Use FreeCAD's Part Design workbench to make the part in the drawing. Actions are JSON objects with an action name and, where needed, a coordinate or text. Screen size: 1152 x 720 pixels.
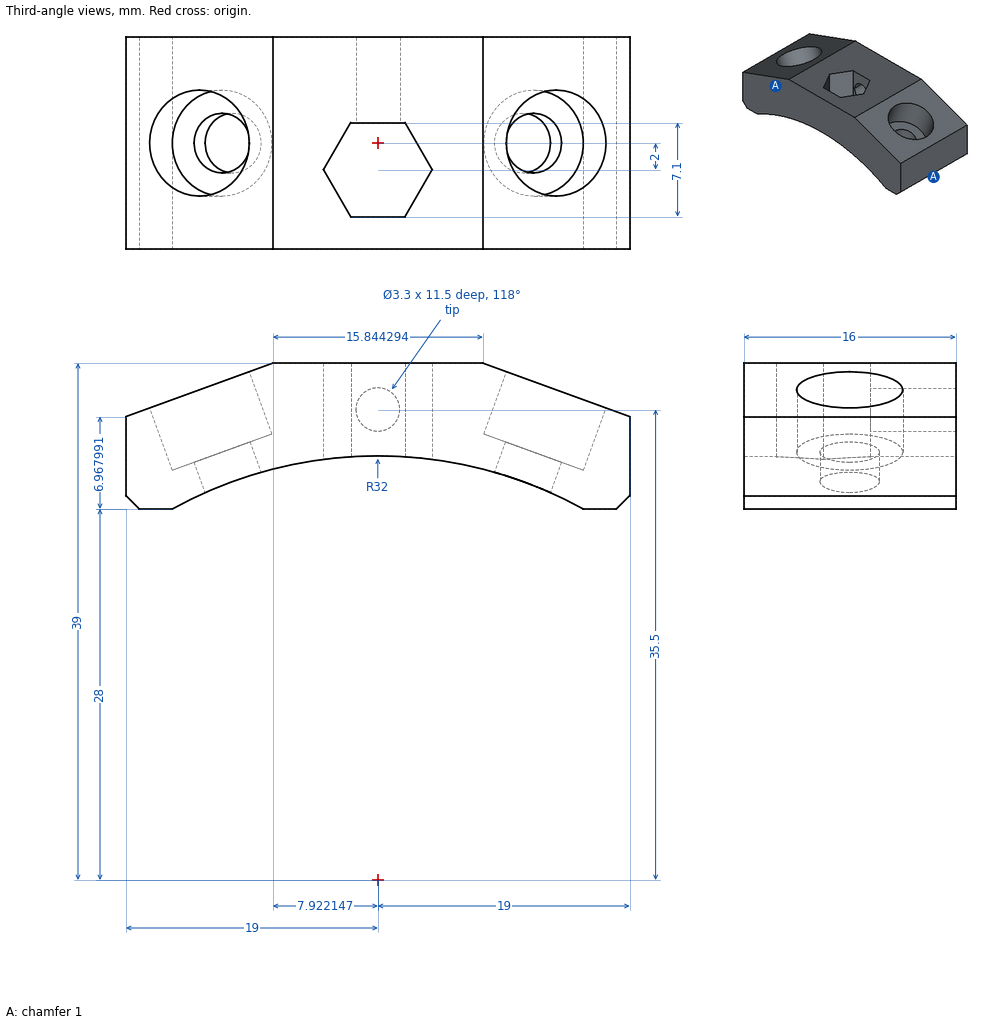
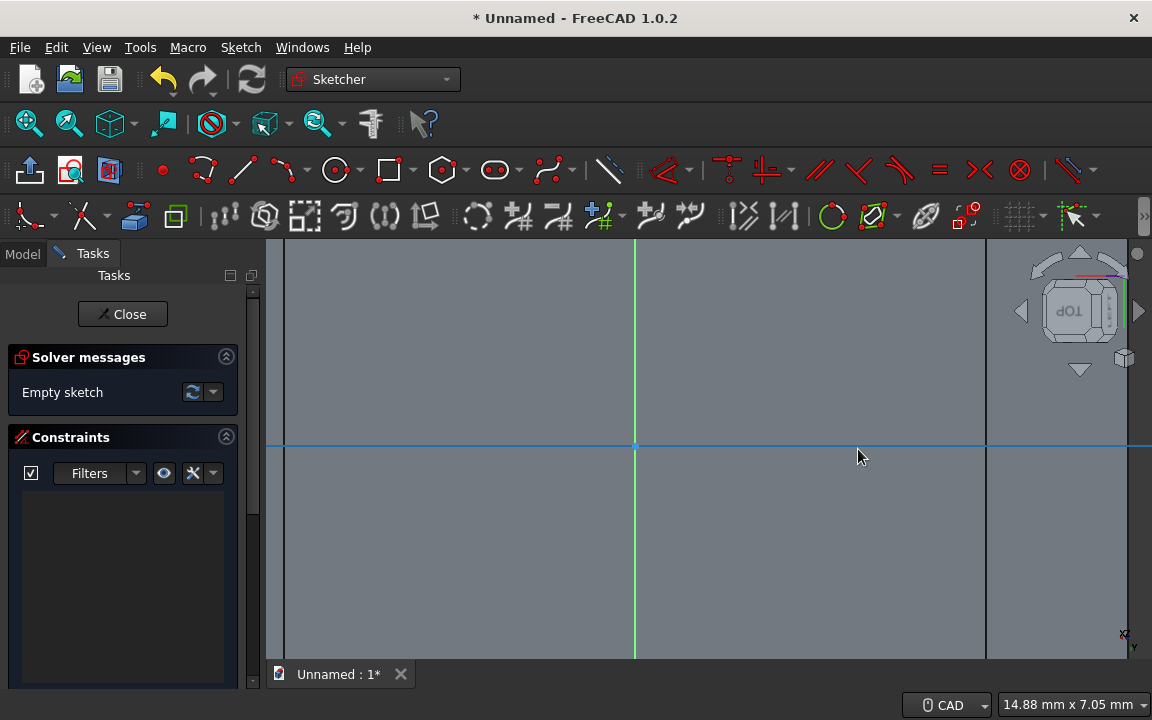
{"action": "key", "text": "g c"}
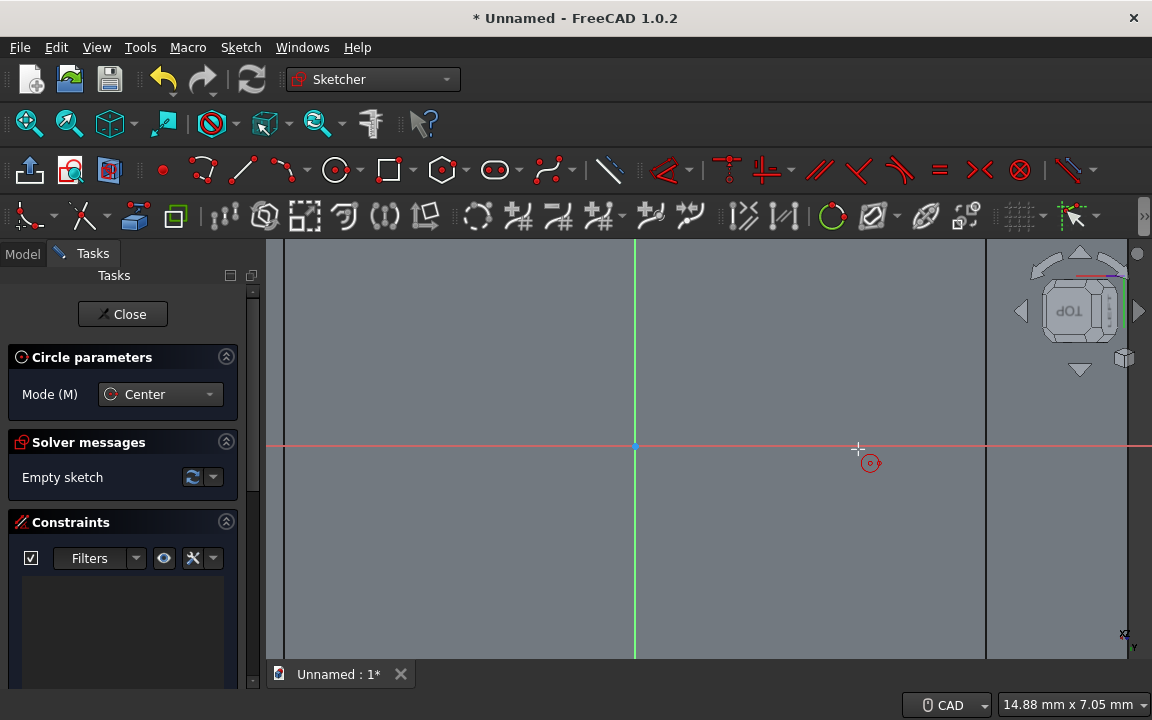
{"action": "left_click", "coordinate": [635, 446]}
{"action": "left_click", "coordinate": [730, 352]}
{"action": "key", "text": "Escape"}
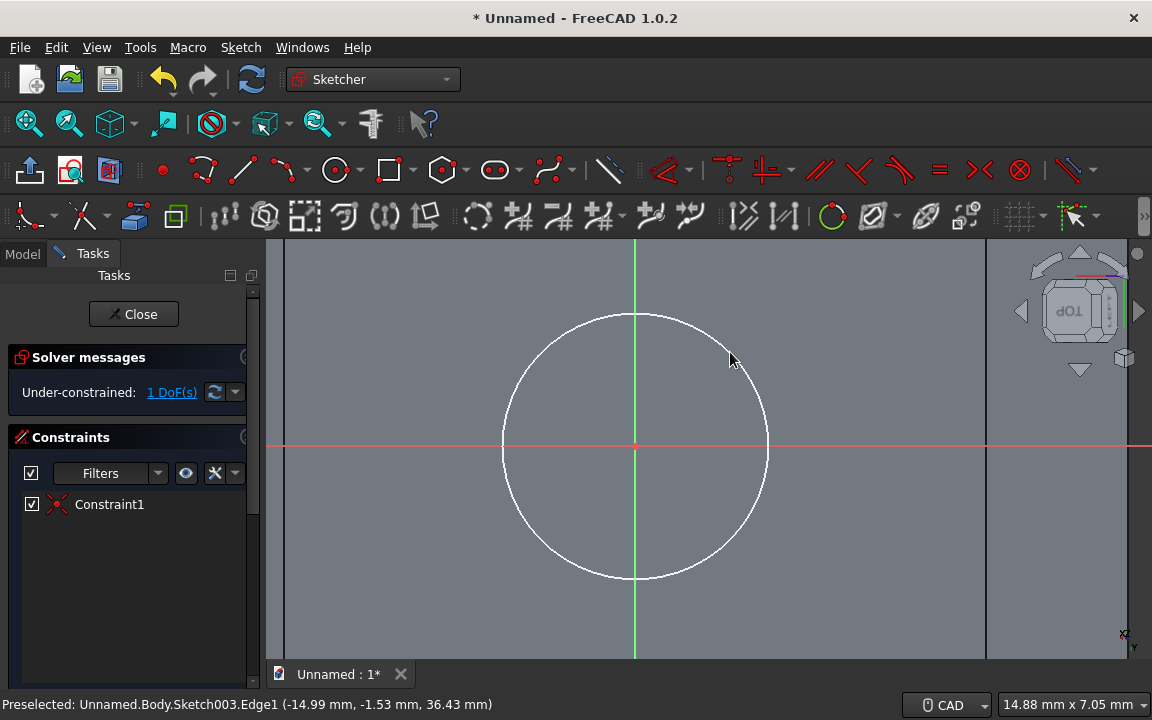
{"action": "key", "text": "d"}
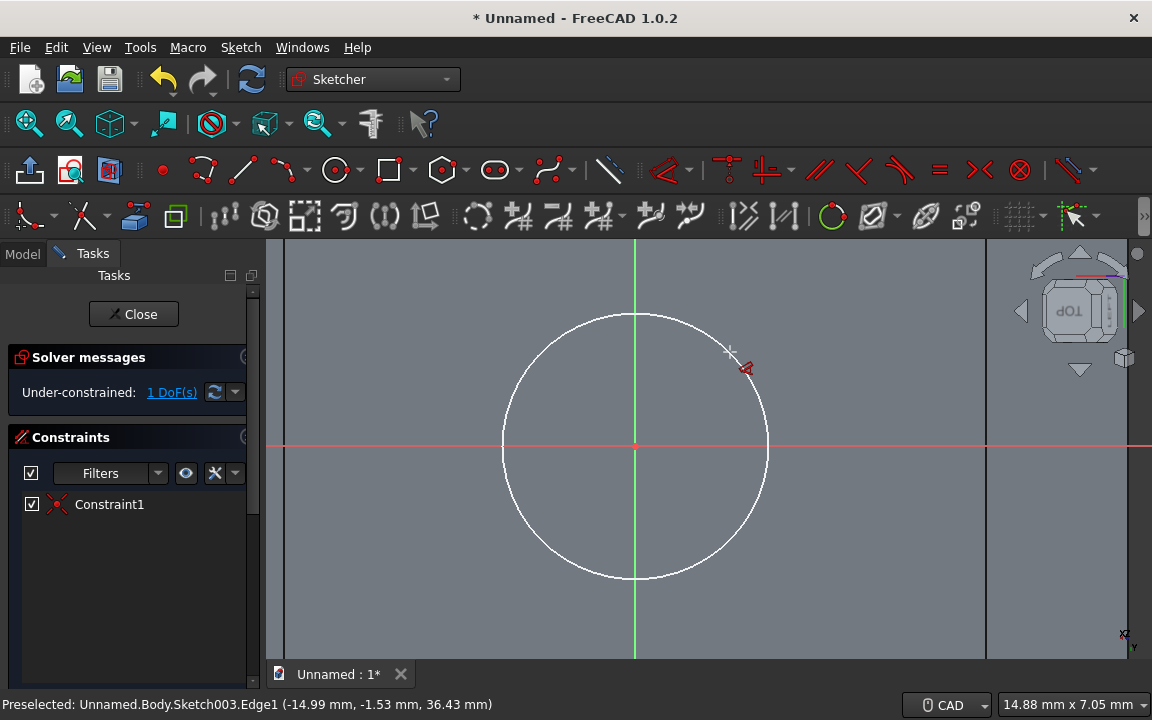
{"action": "left_click", "coordinate": [729, 352]}
{"action": "left_click", "coordinate": [752, 329]}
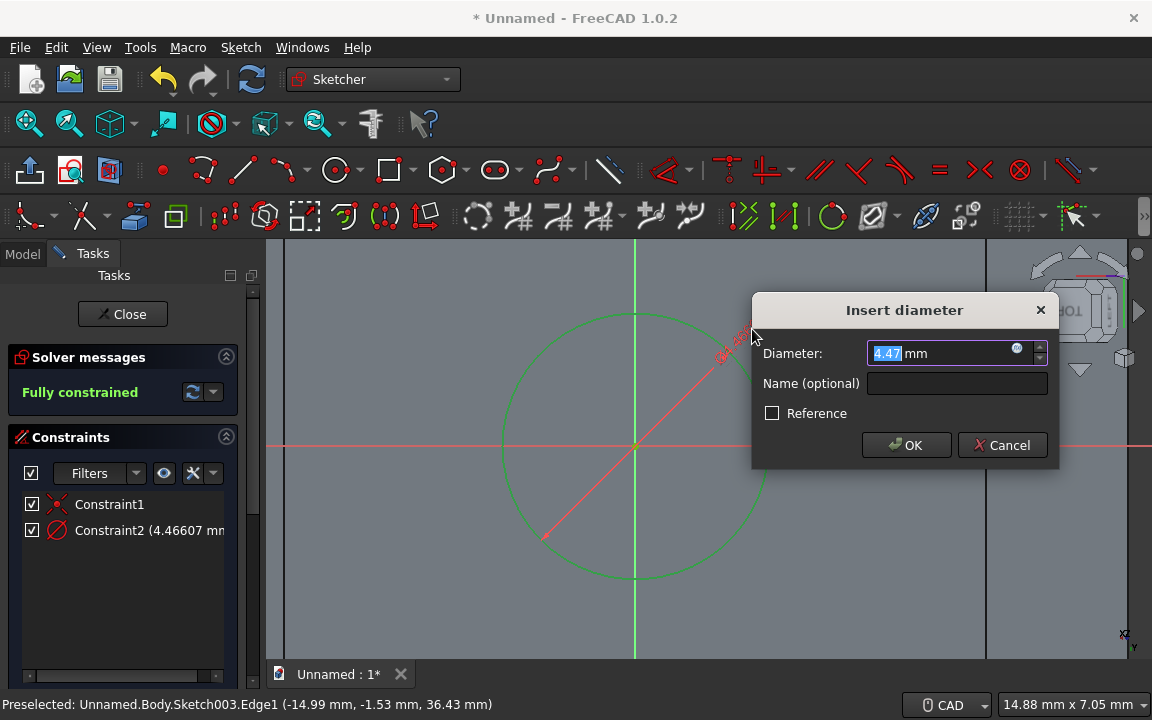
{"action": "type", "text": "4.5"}
{"action": "key", "text": "Return"}
{"action": "key", "text": "Escape"}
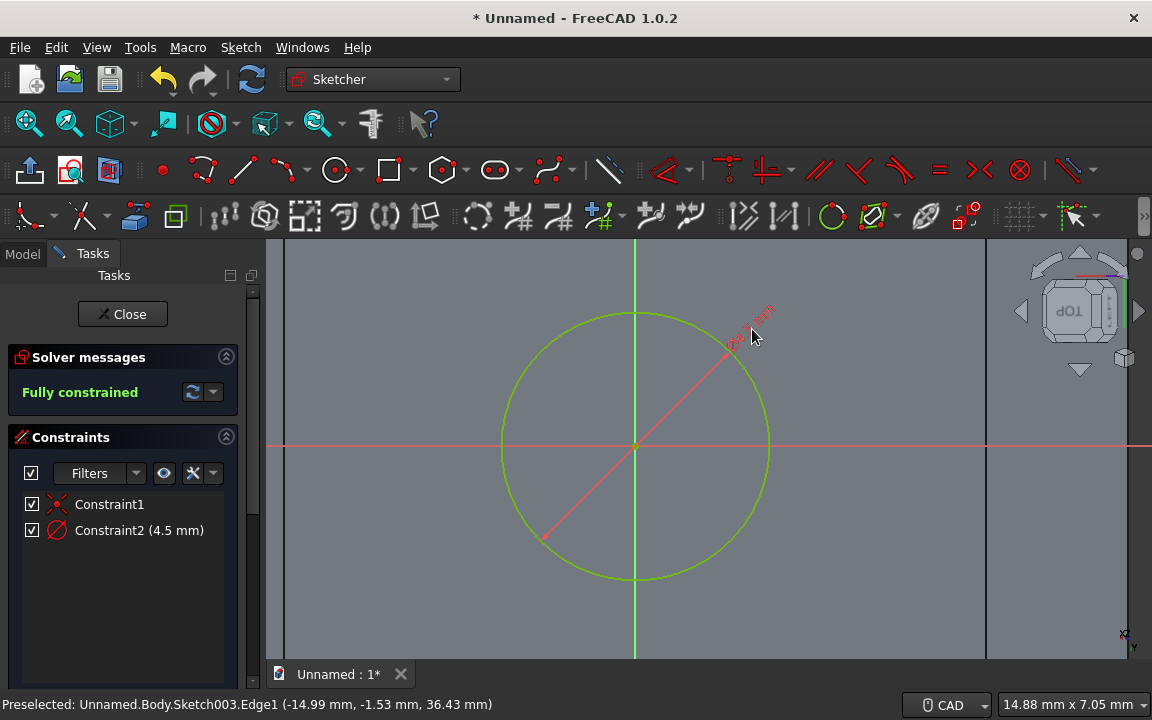
{"action": "left_click", "coordinate": [123, 314]}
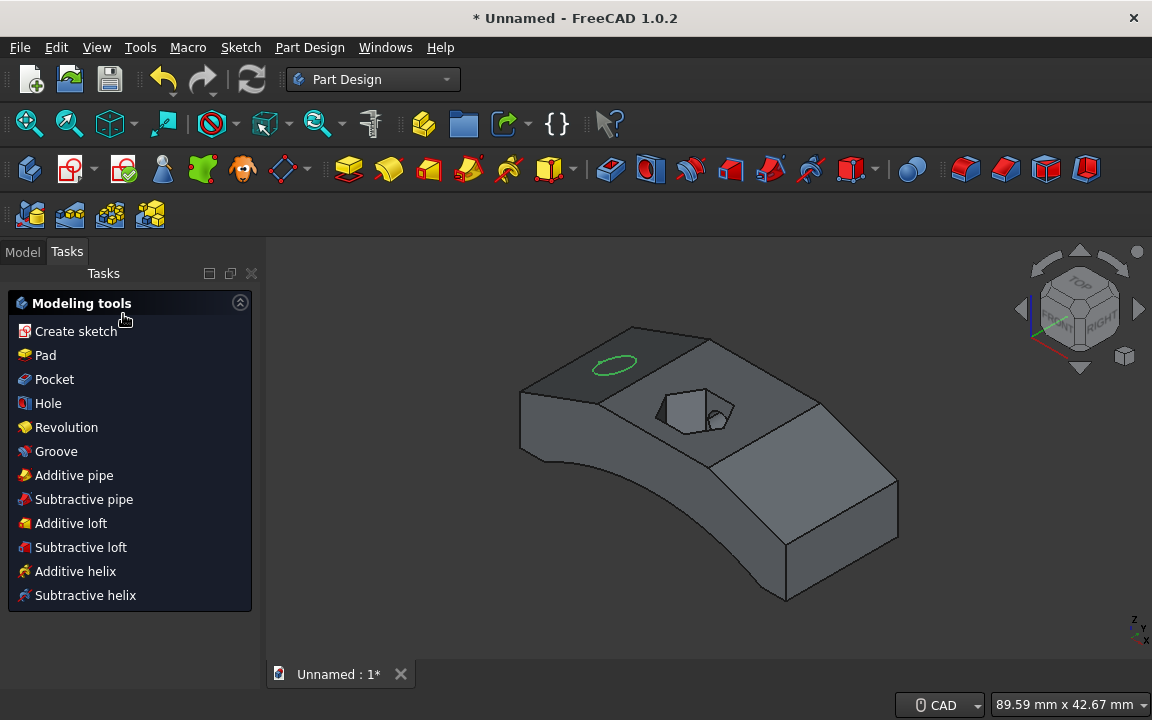
{"action": "left_click", "coordinate": [652, 170]}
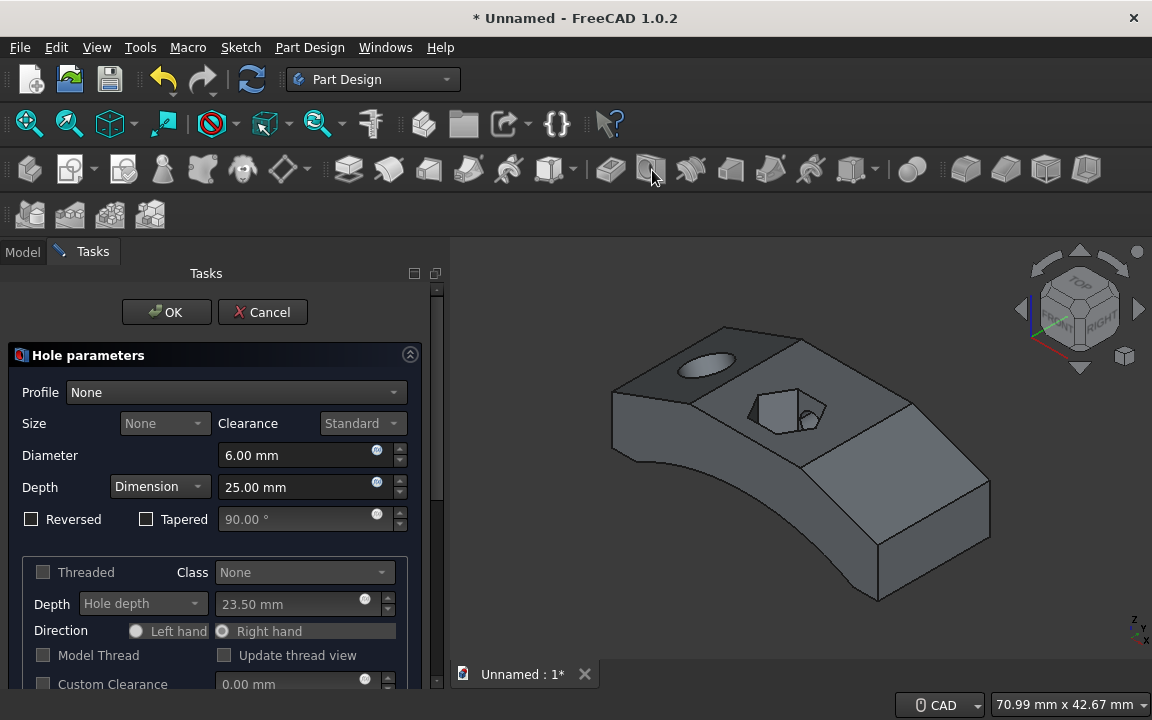
{"action": "triple_click", "coordinate": [305, 455]}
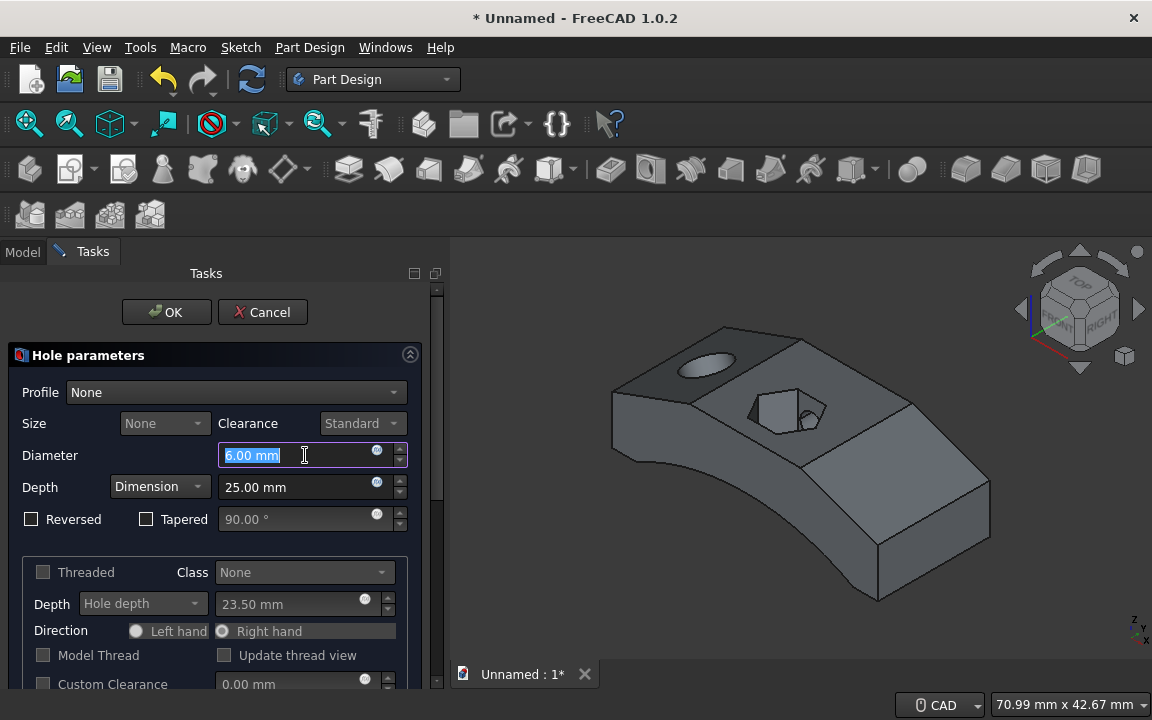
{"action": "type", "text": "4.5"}
{"action": "key", "text": "Tab"}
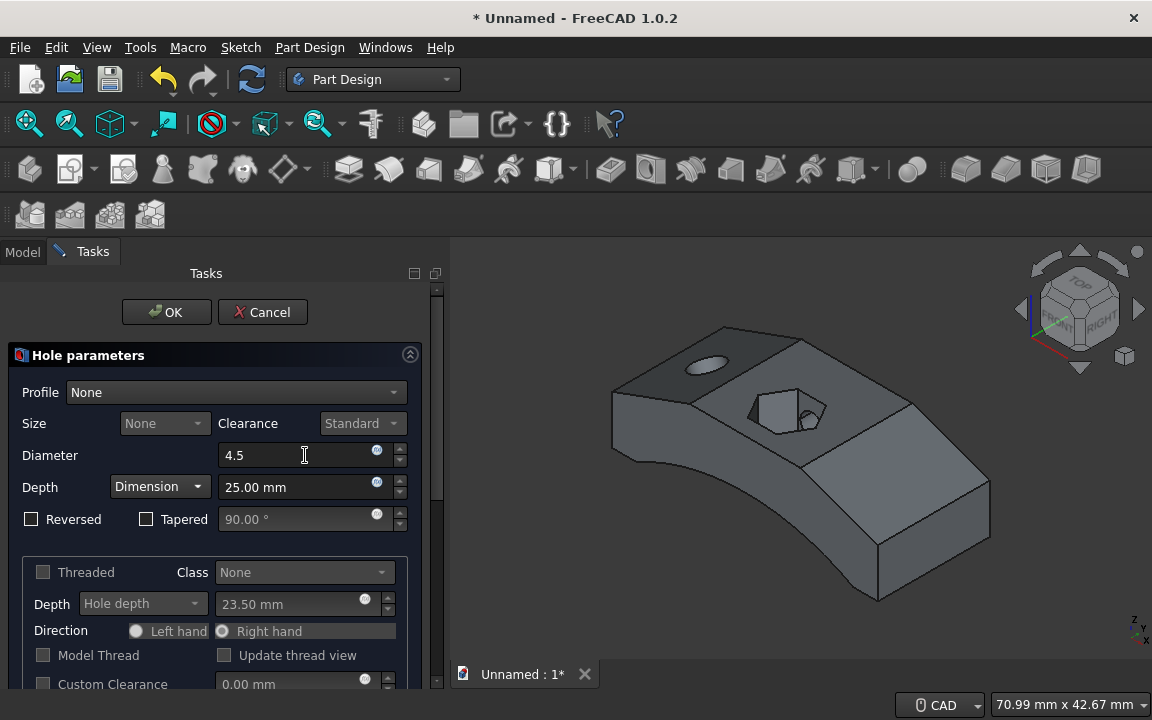
{"action": "left_click", "coordinate": [161, 486]}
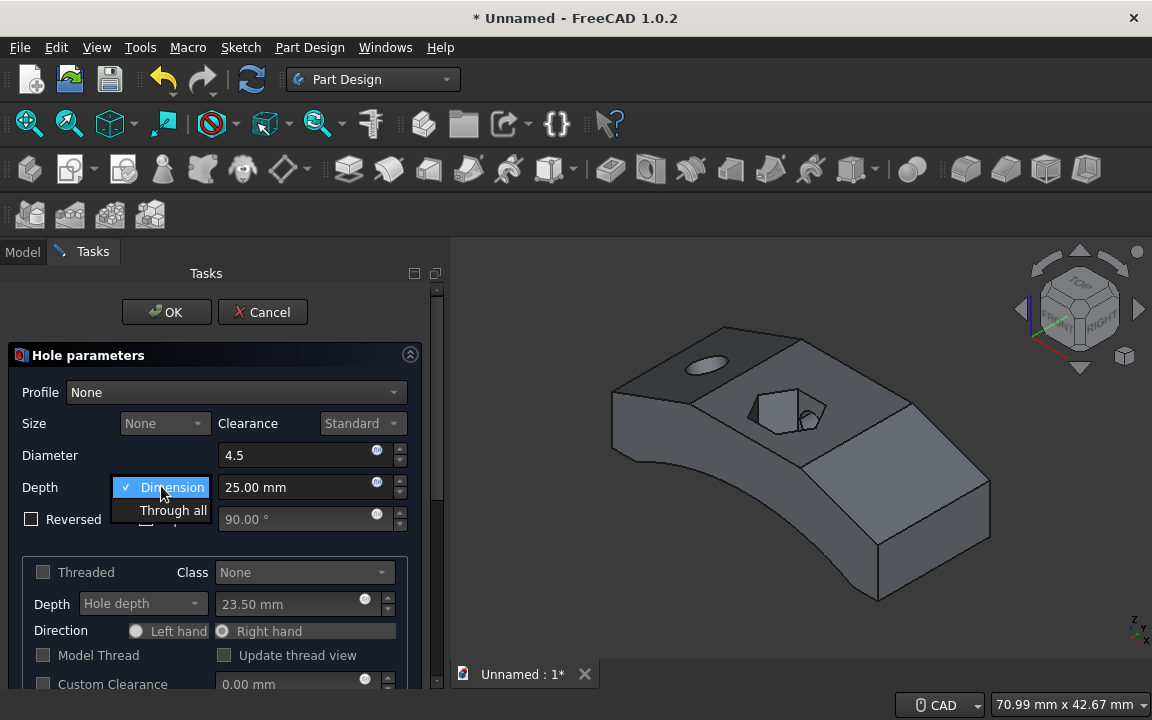
{"action": "left_click", "coordinate": [160, 510]}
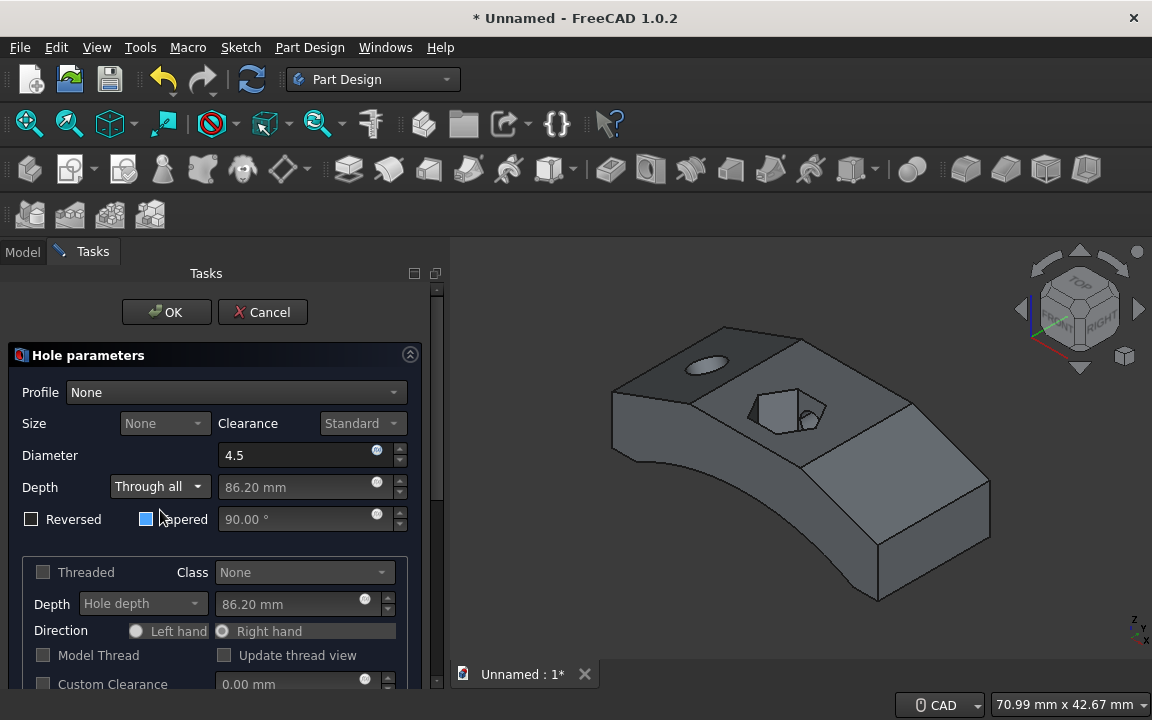
{"action": "scroll", "coordinate": [437, 486], "scroll_direction": "down", "scroll_amount": 3}